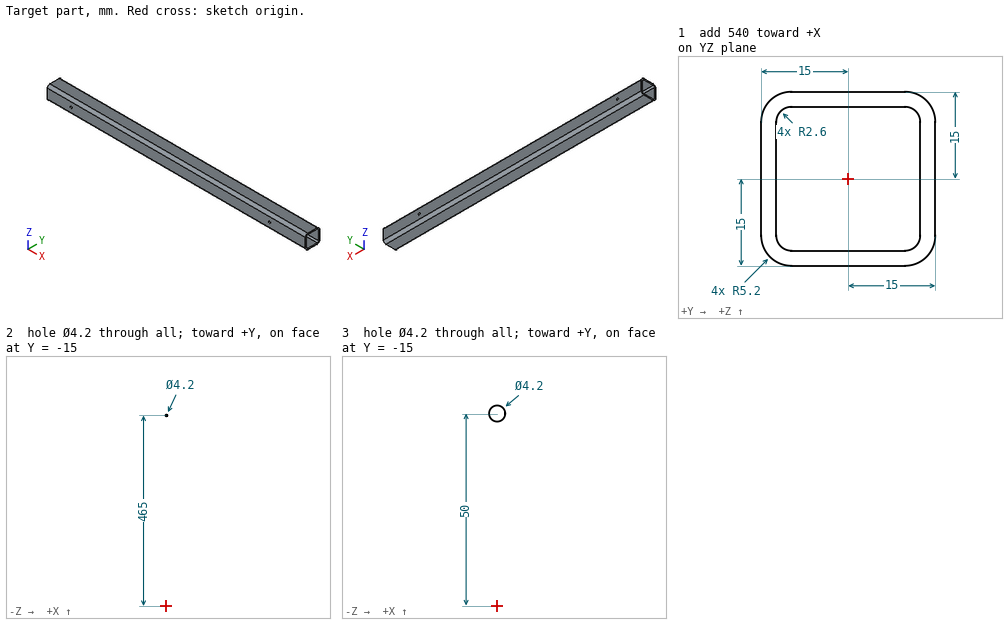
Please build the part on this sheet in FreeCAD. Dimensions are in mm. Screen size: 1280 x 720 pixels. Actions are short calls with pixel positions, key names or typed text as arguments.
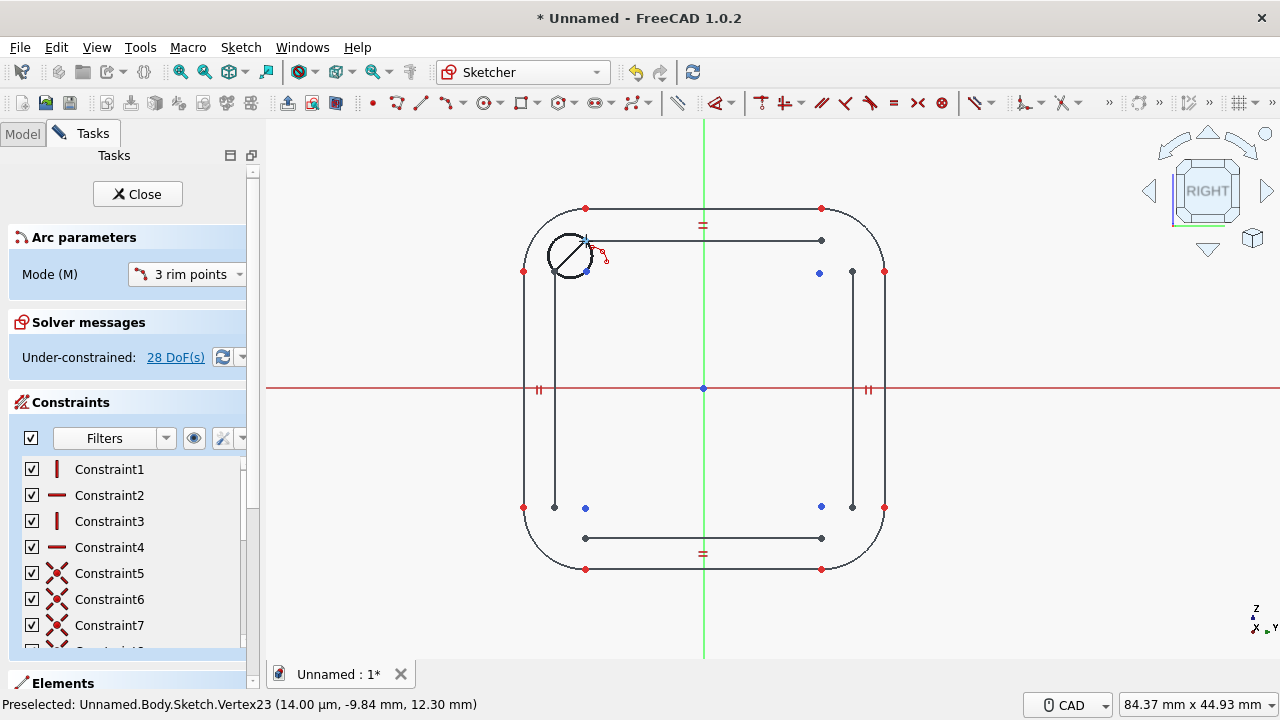
scroll(564, 249, up, 3)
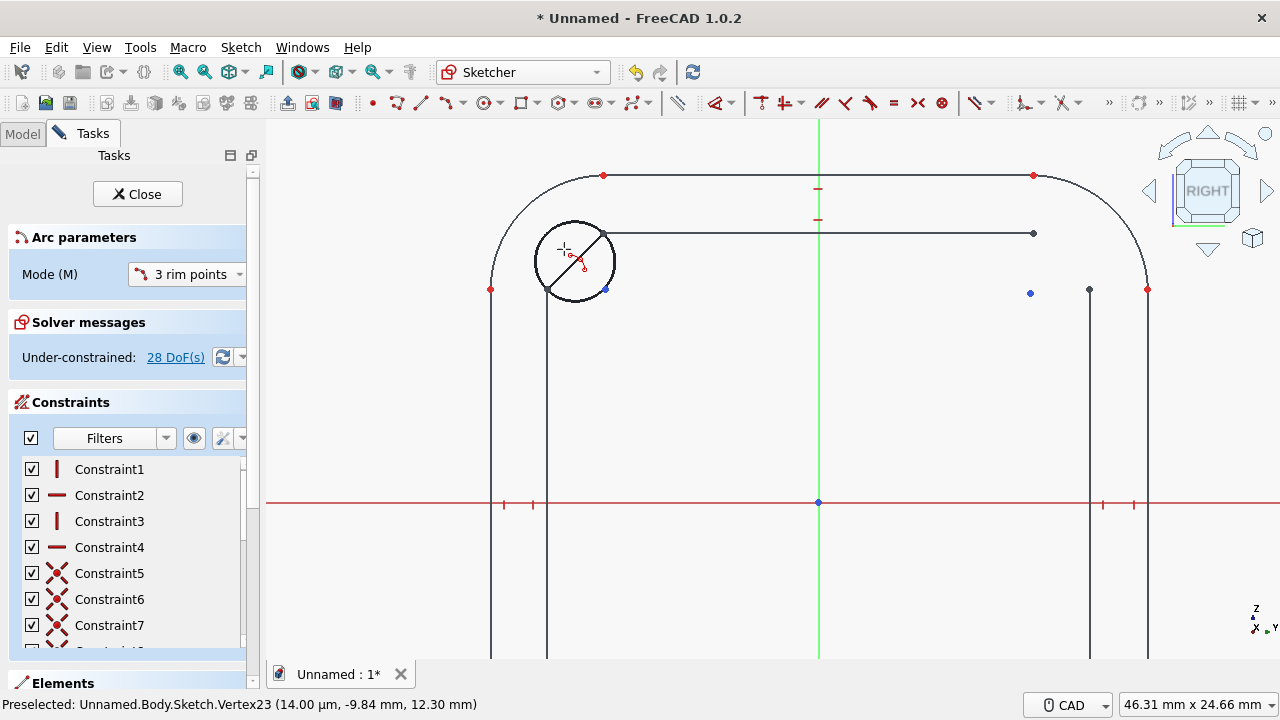
click(564, 248)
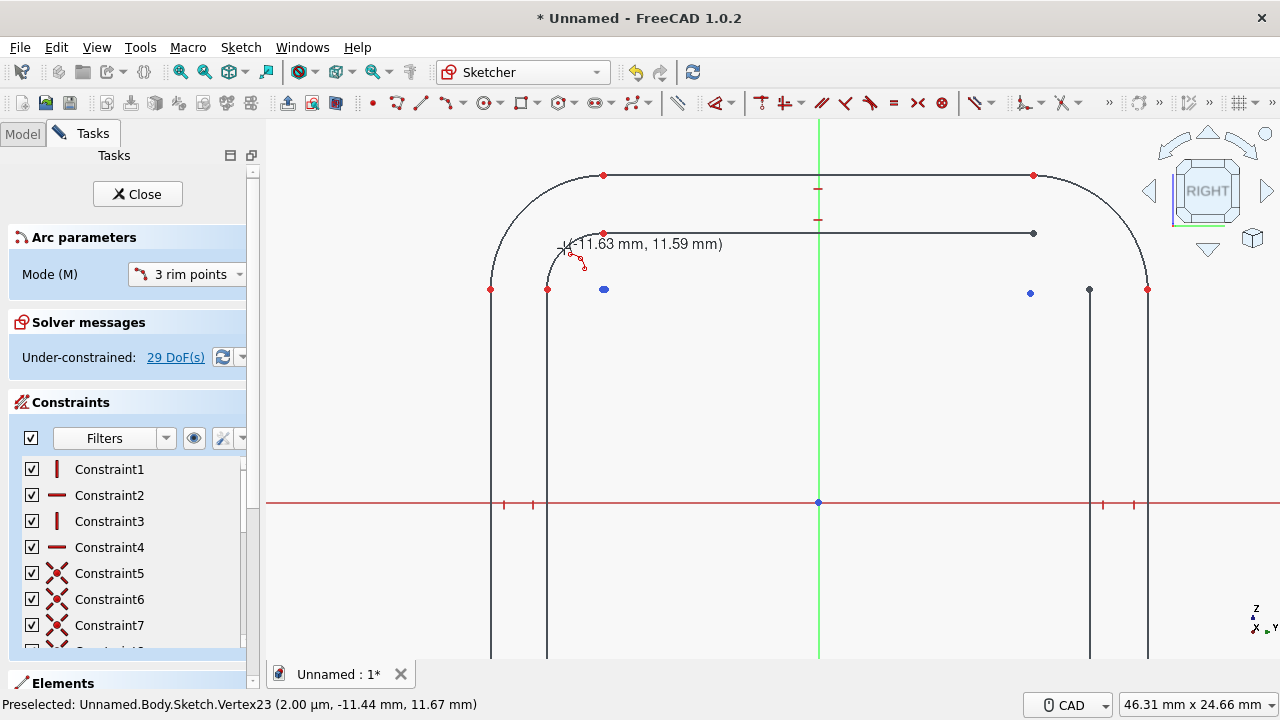
click(1034, 233)
click(1090, 290)
click(1074, 248)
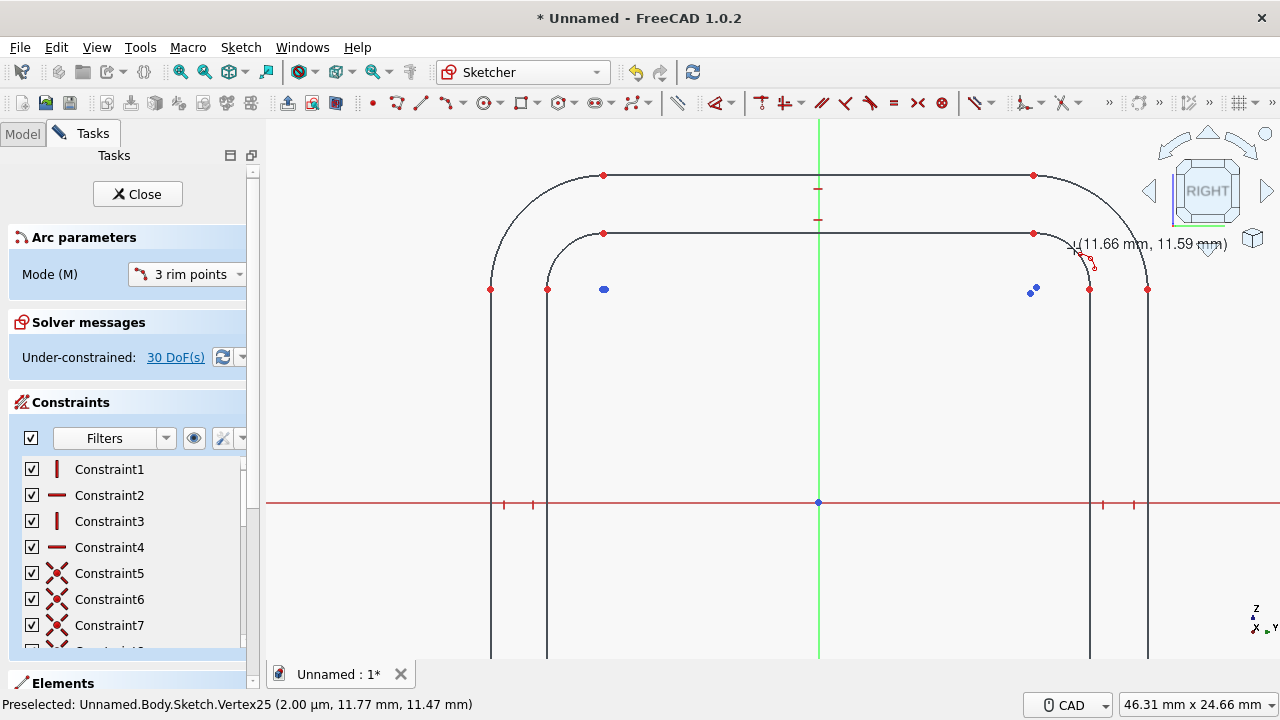
scroll(566, 251, down, 3)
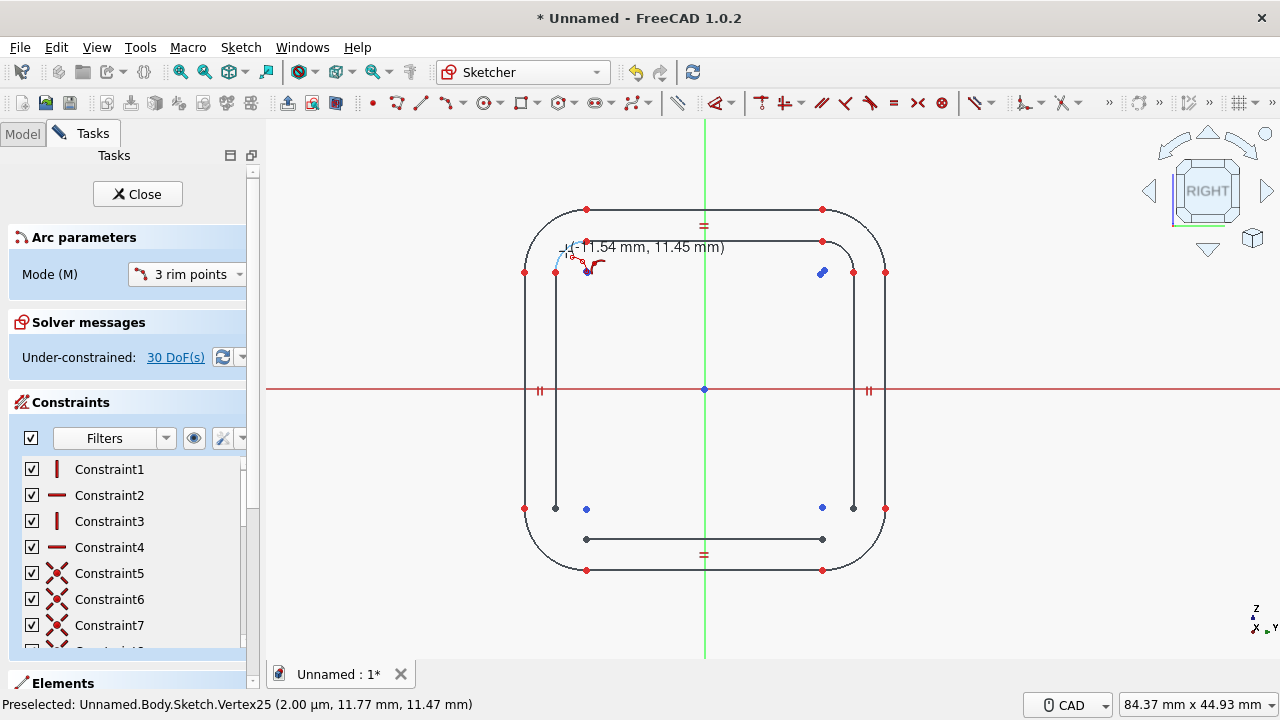
click(854, 508)
click(823, 539)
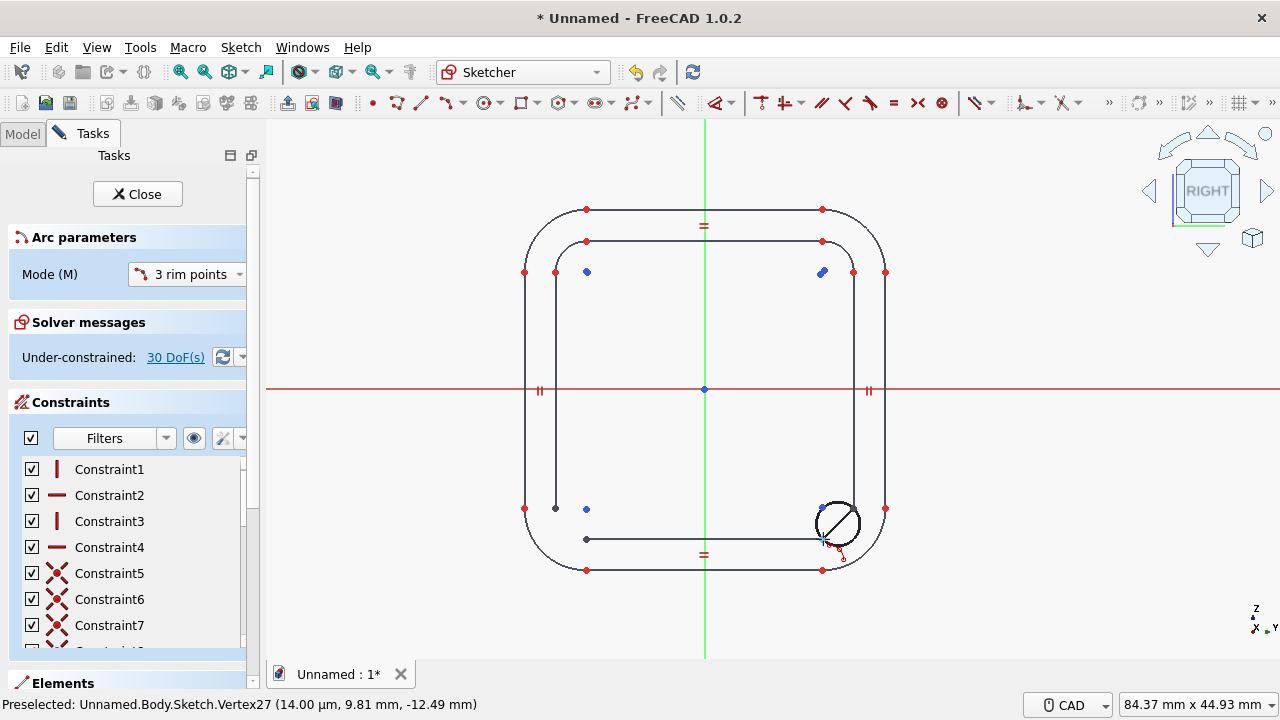
scroll(845, 529, up, 3)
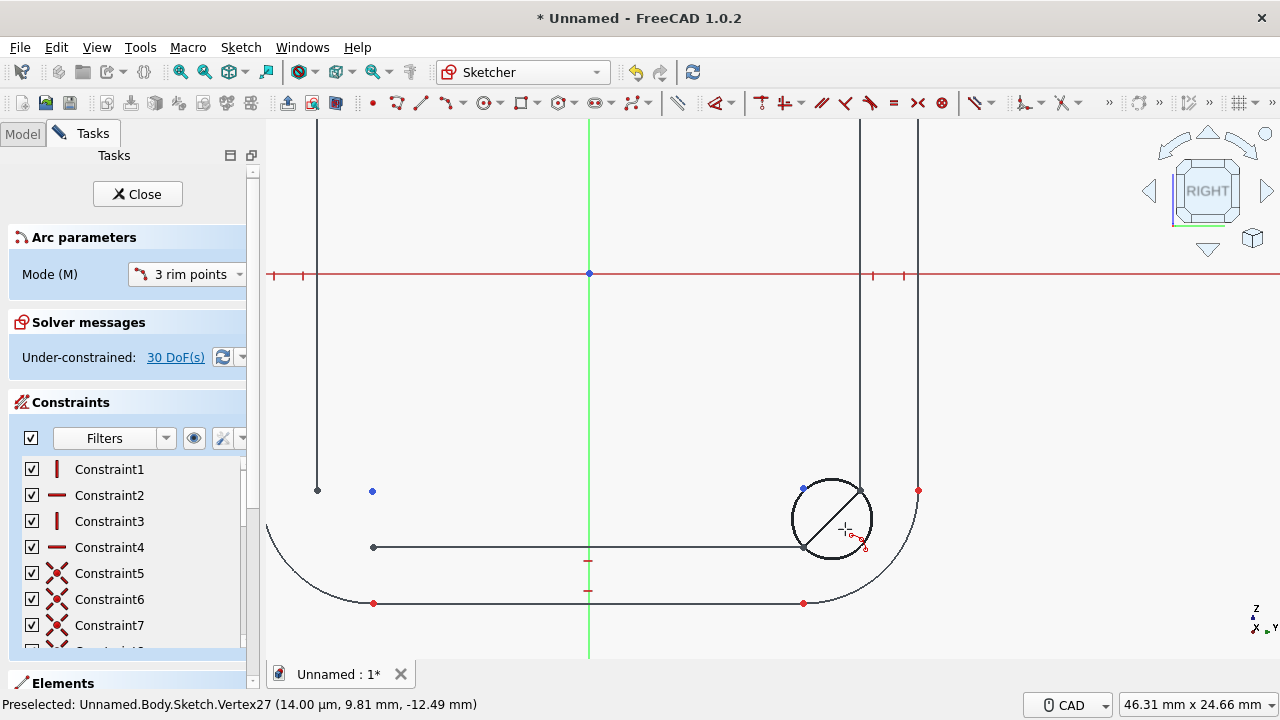
click(844, 529)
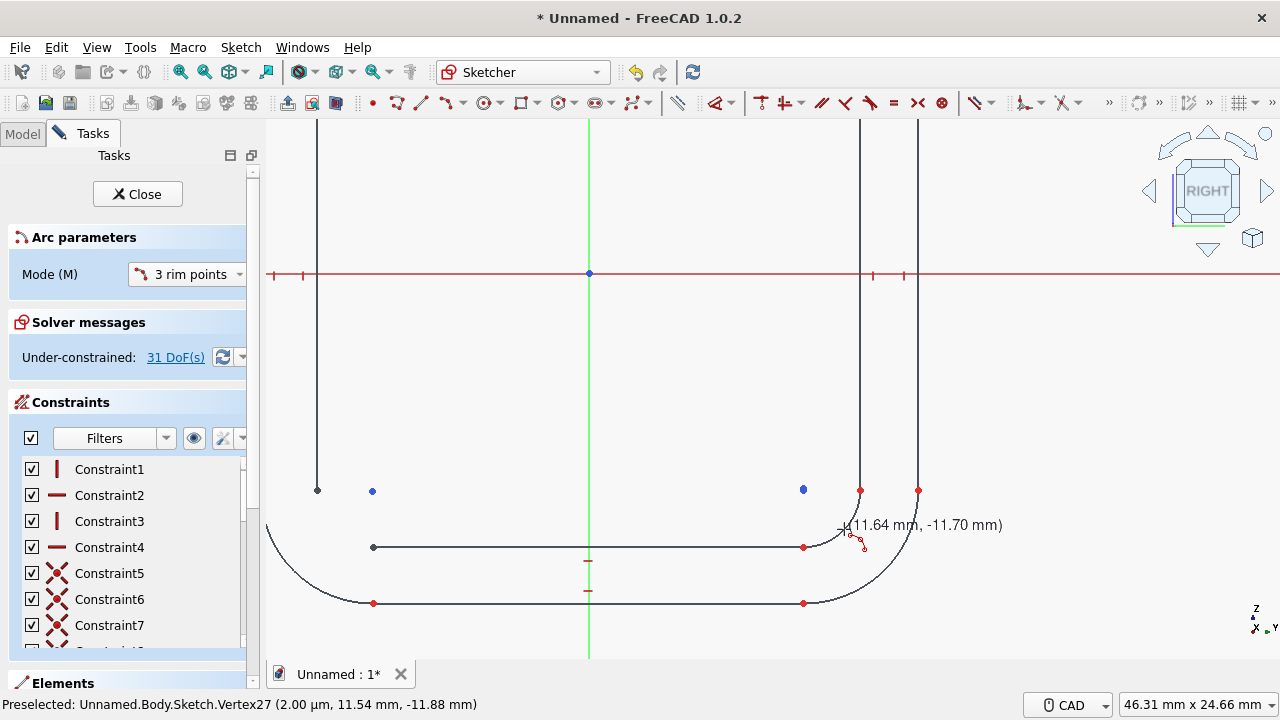
click(374, 547)
click(317, 491)
click(334, 529)
key(Escape)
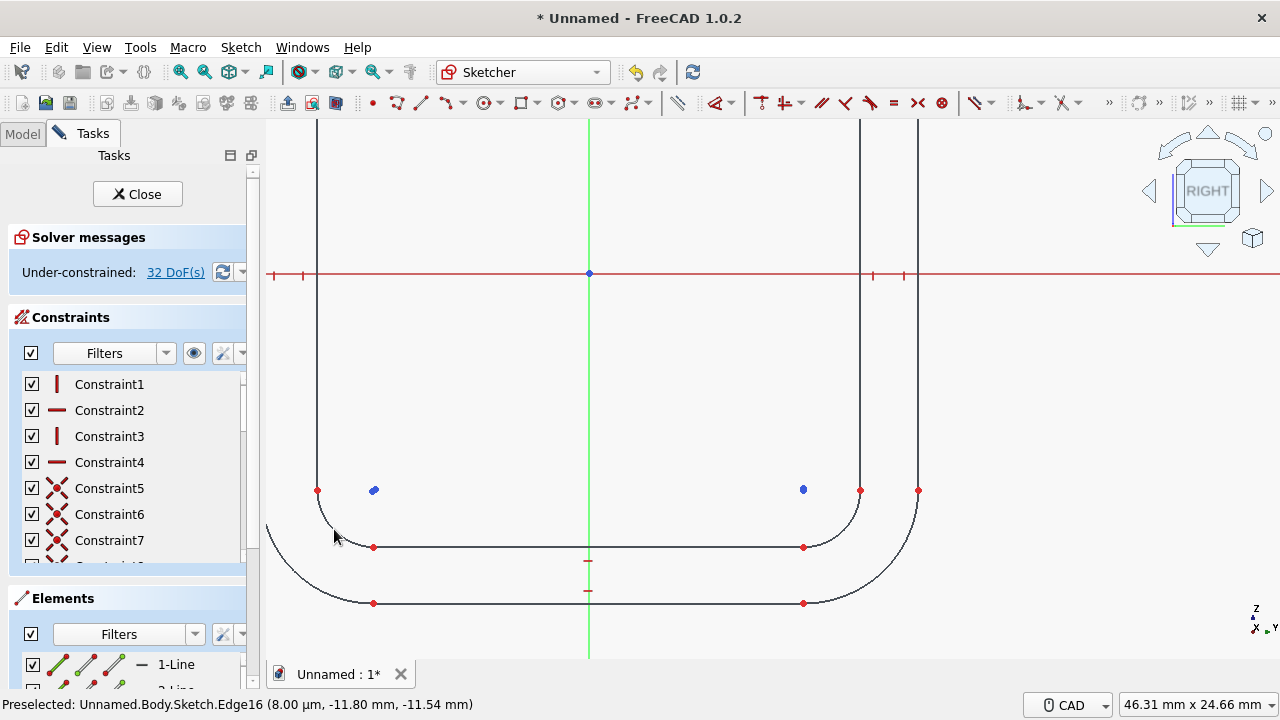
scroll(845, 529, down, 3)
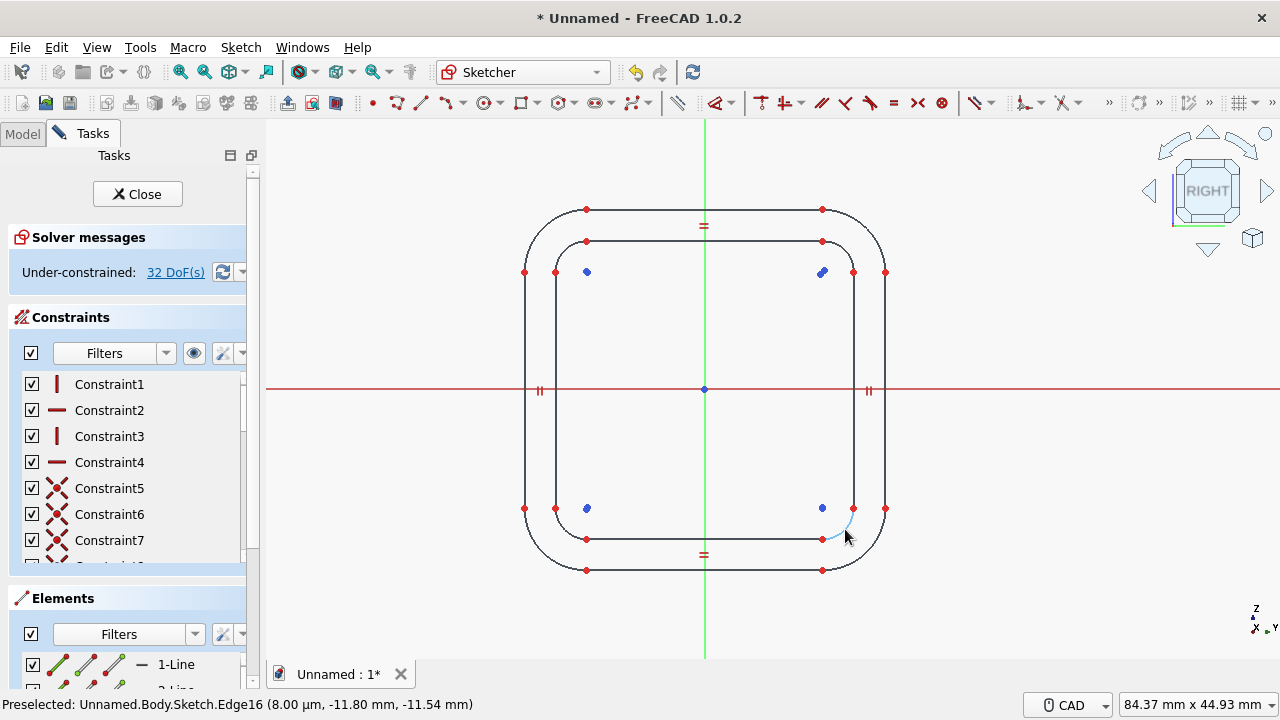
click(525, 343)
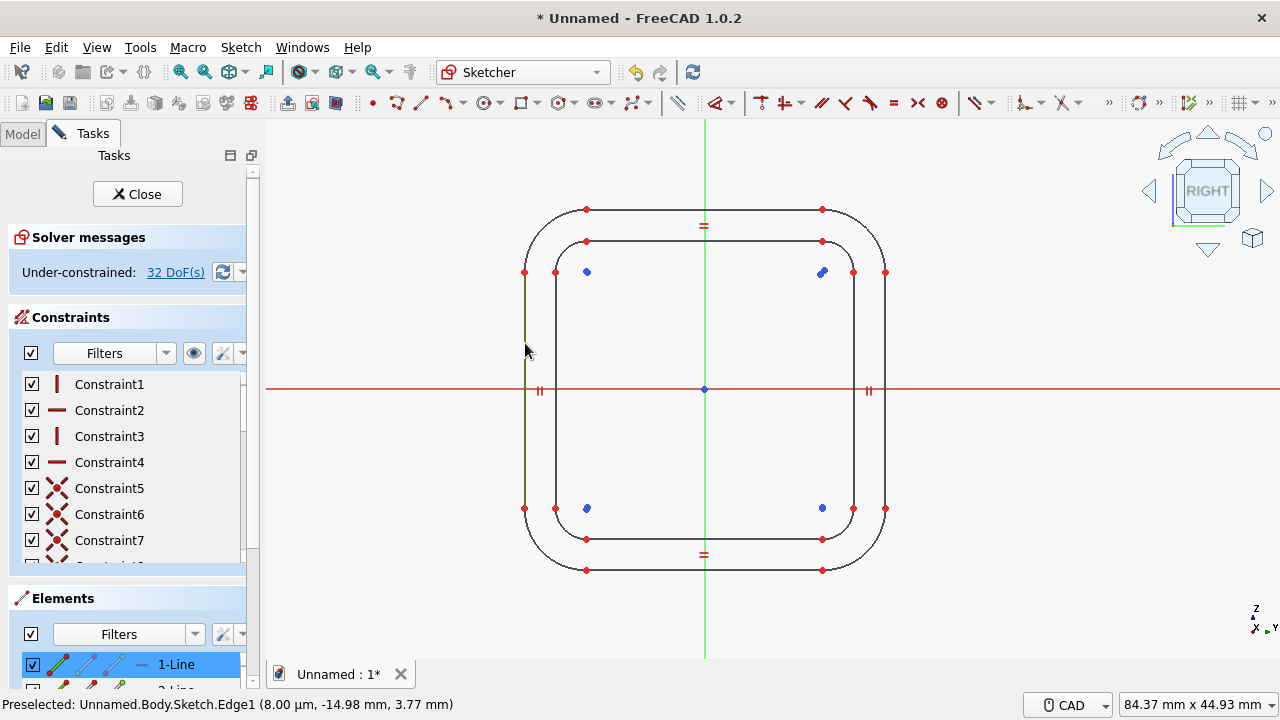
click(531, 537)